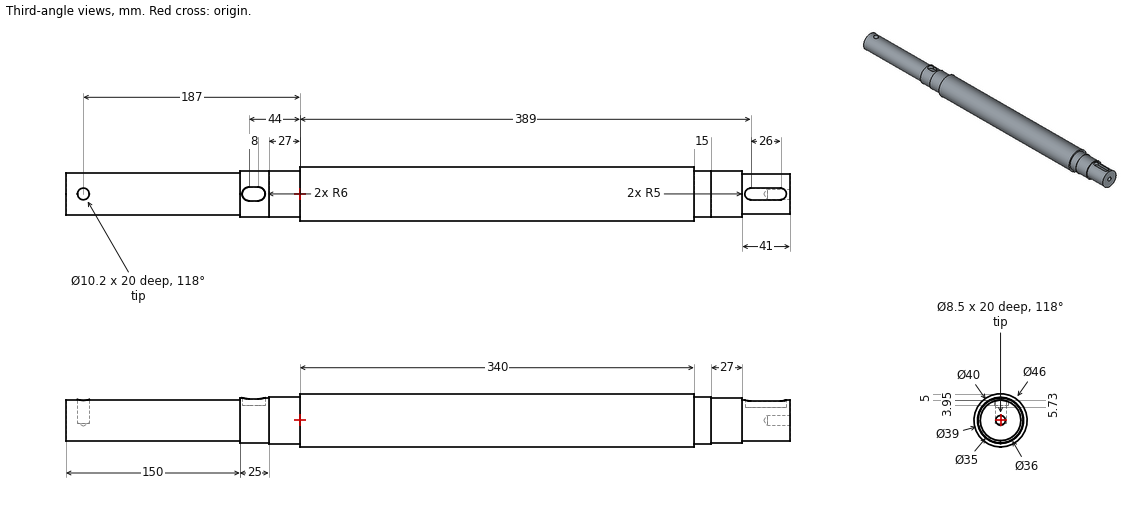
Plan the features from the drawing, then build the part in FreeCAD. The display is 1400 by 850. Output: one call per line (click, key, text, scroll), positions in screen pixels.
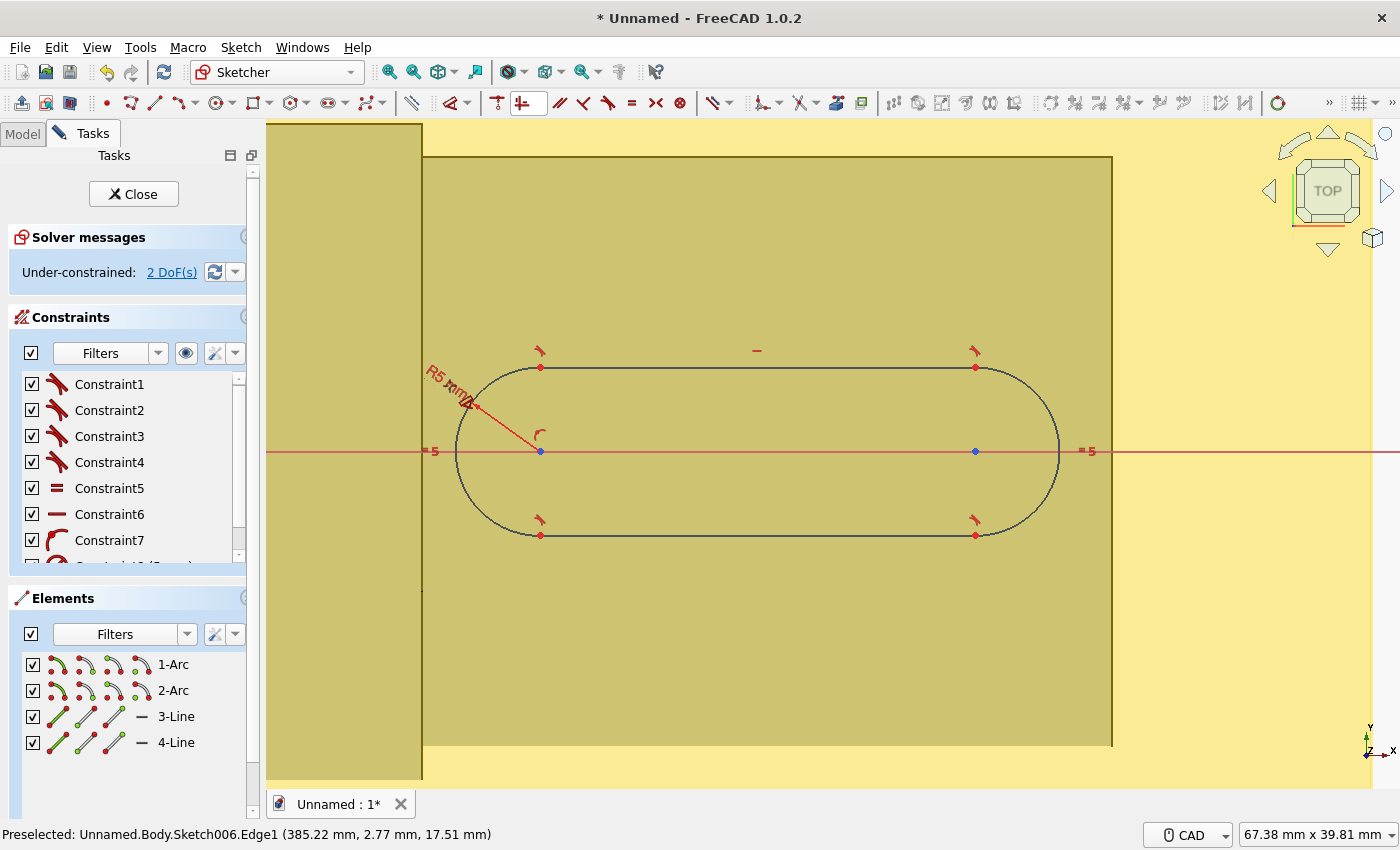
click(671, 368)
click(758, 334)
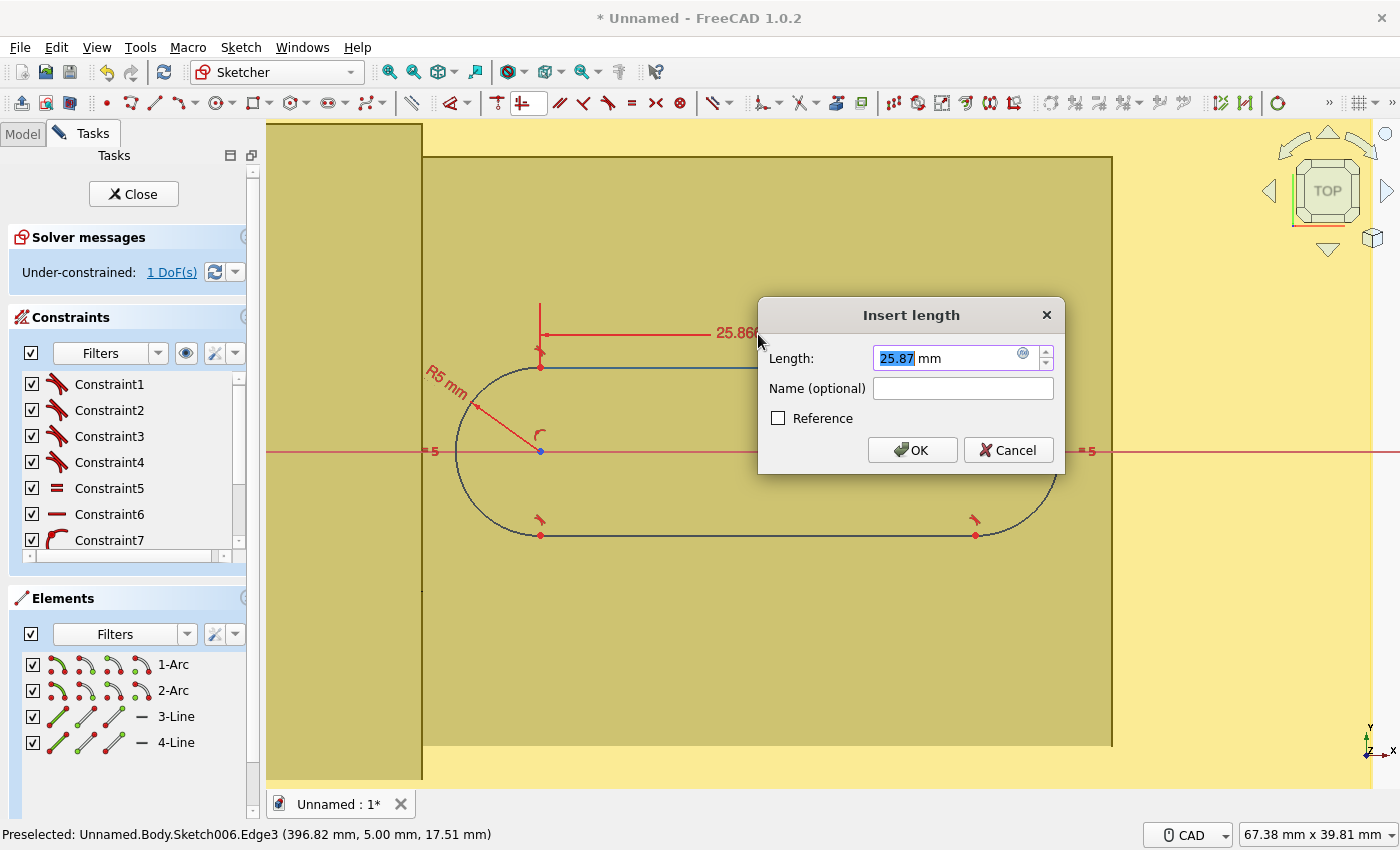
text(26)
key(Return)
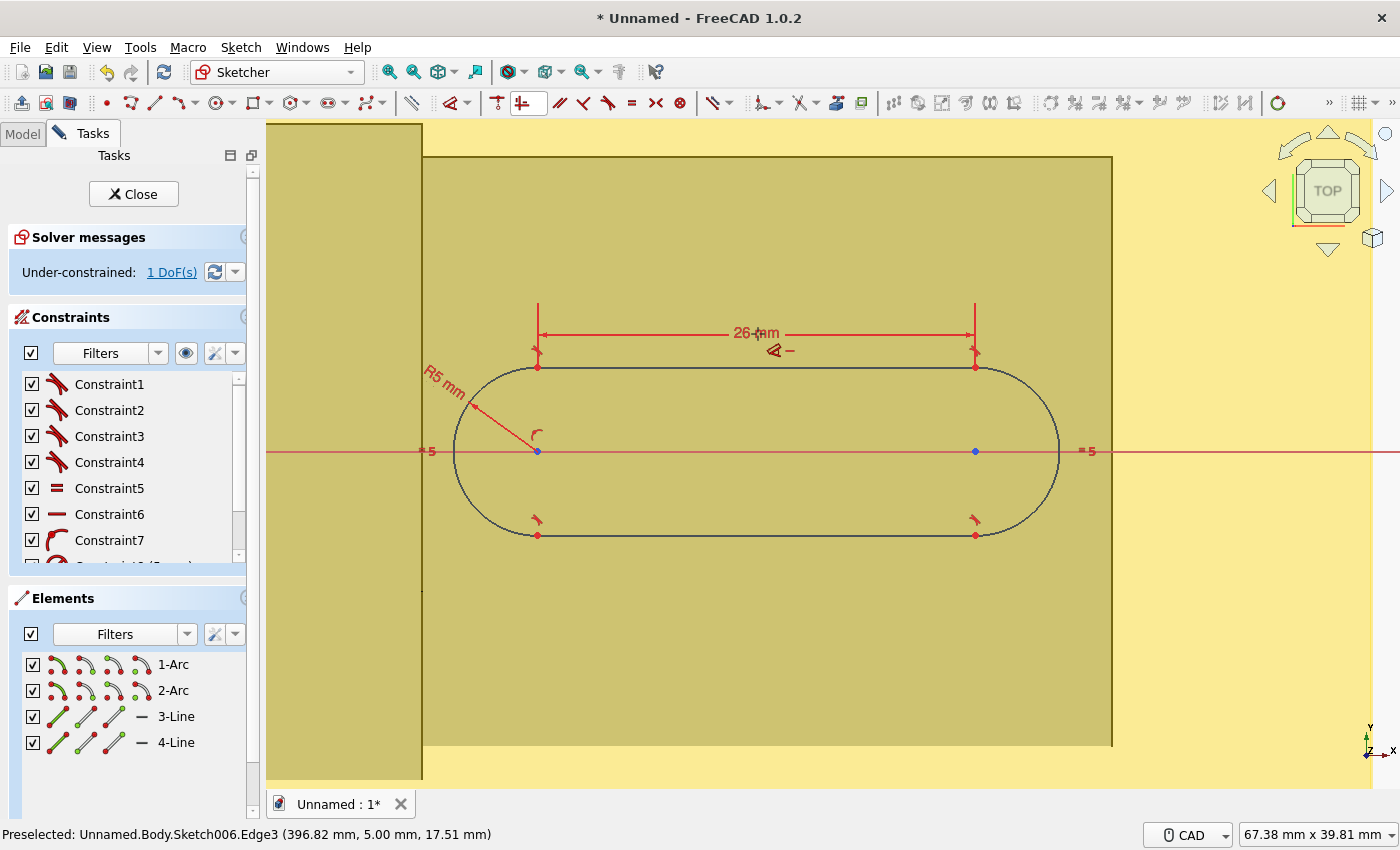
click(538, 368)
click(416, 334)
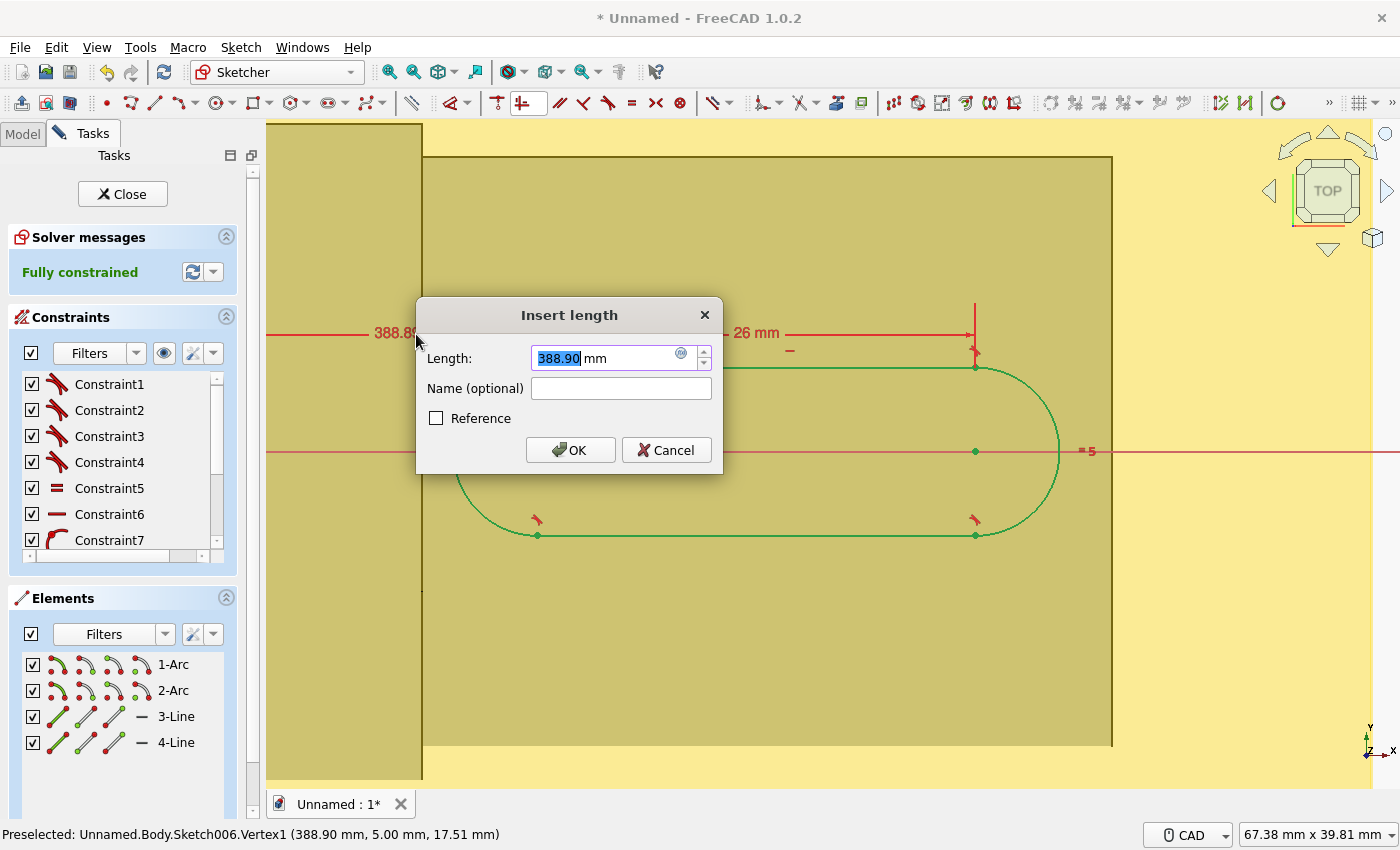
text(389)
key(Return)
key(Escape)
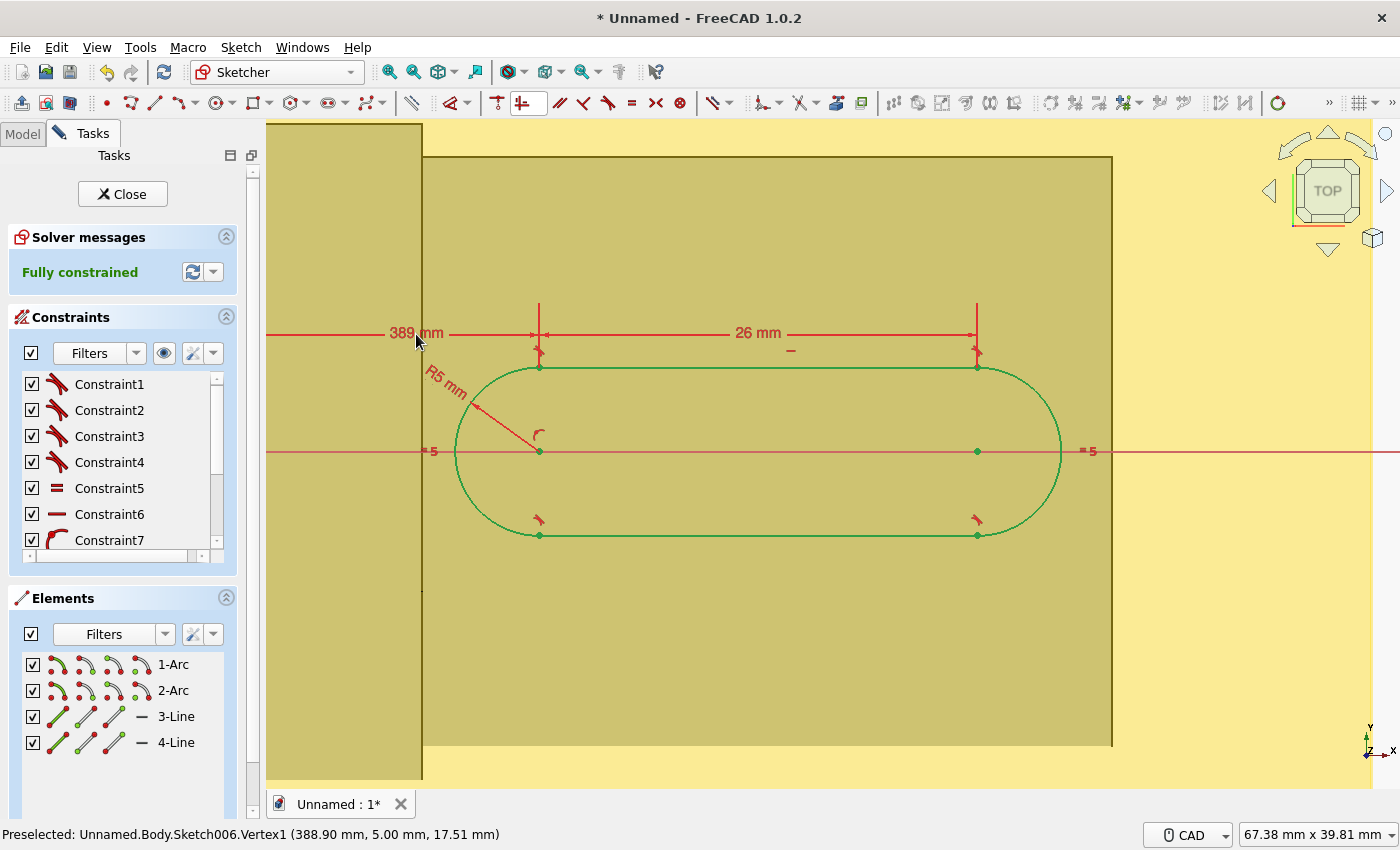
click(123, 194)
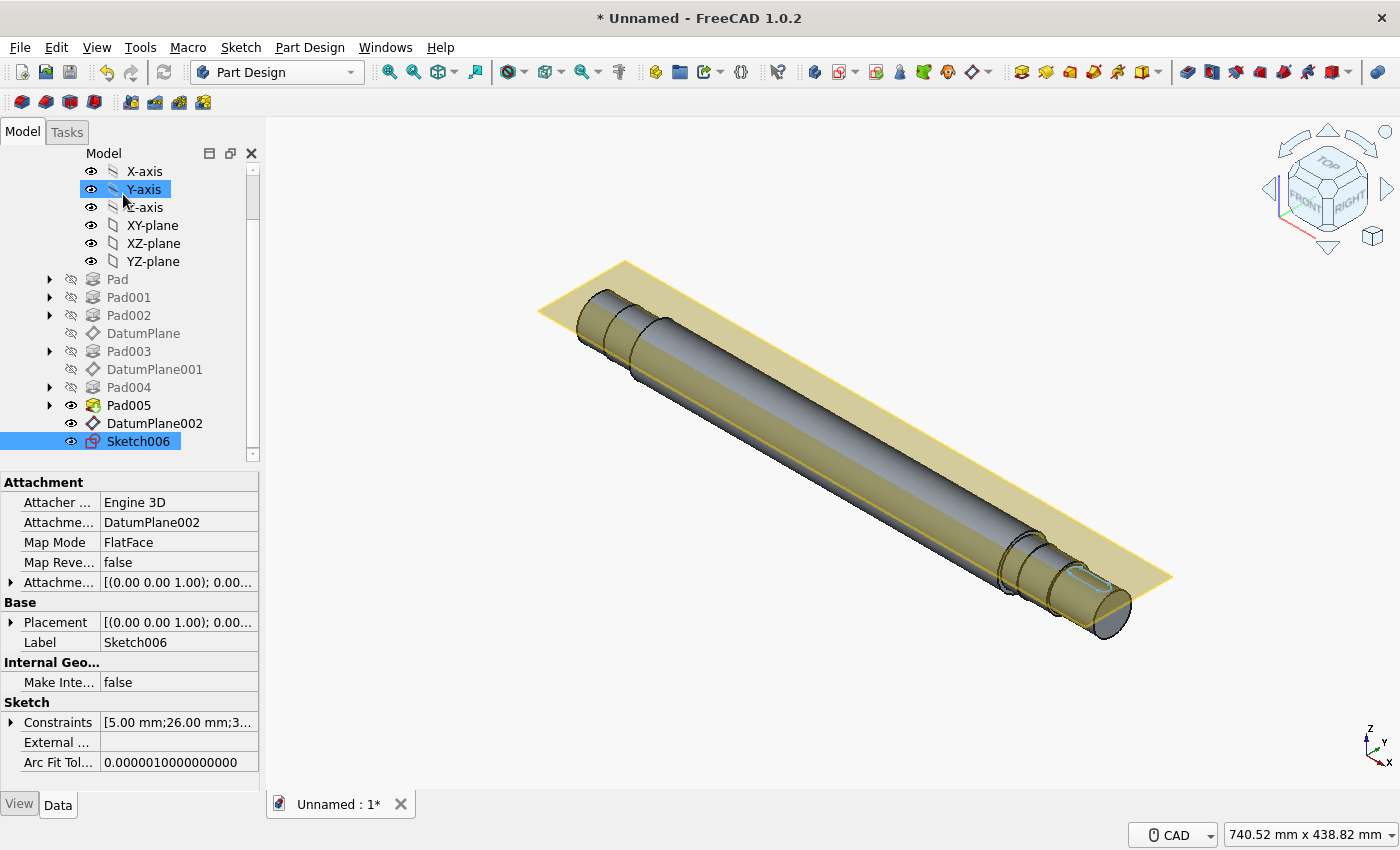
click(1188, 72)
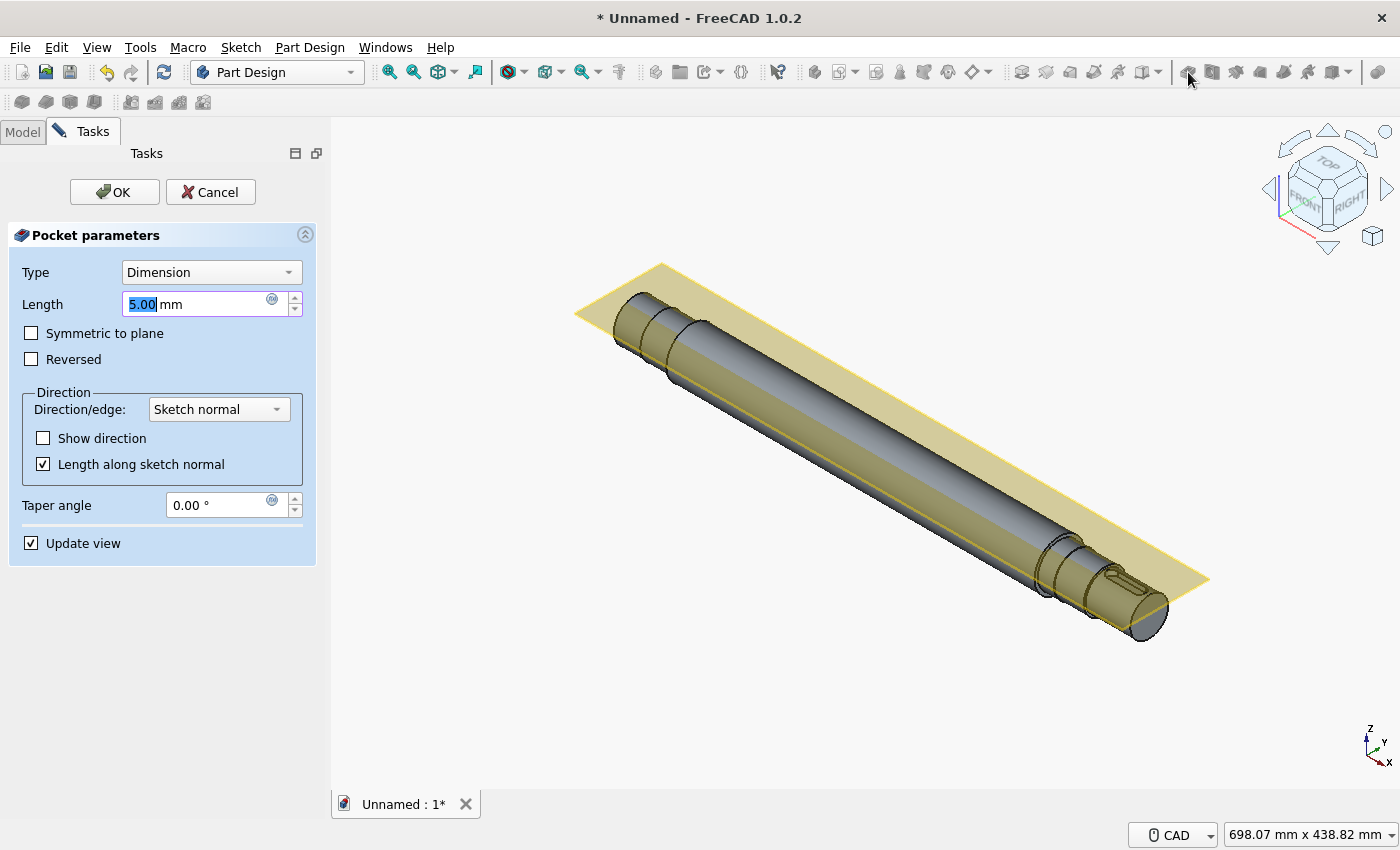
text(5.73)
key(Tab)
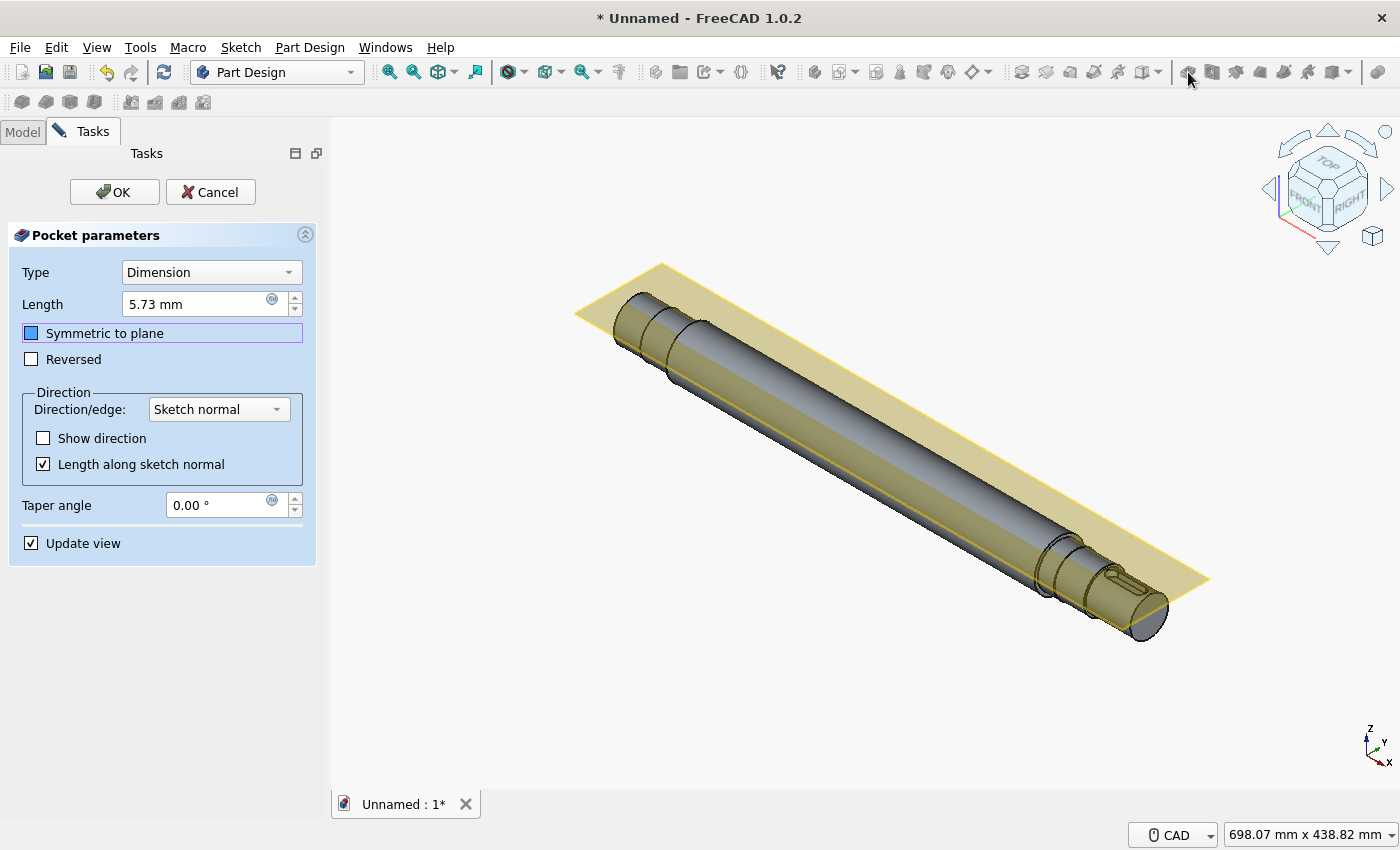
click(115, 192)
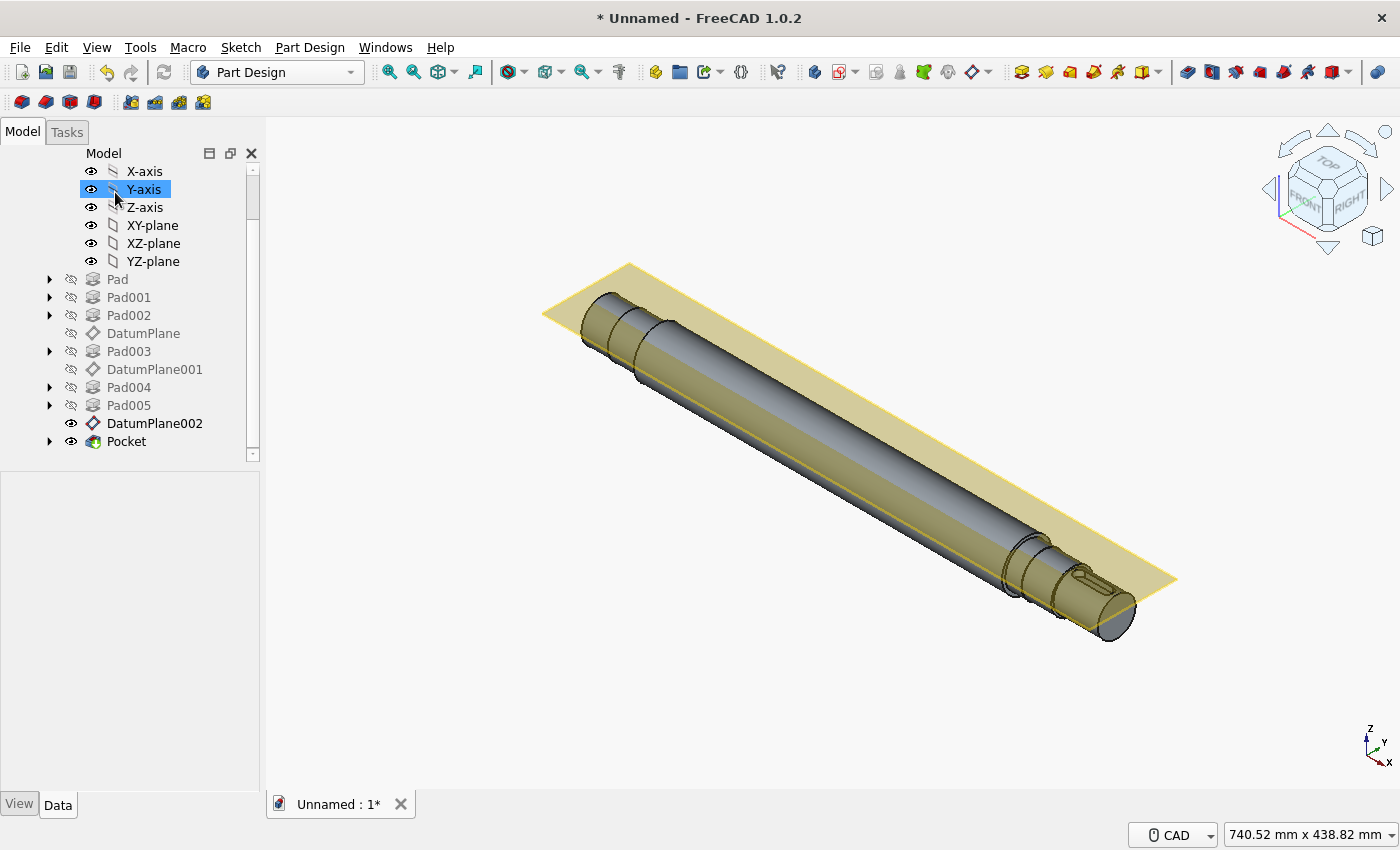
click(116, 423)
key(space)